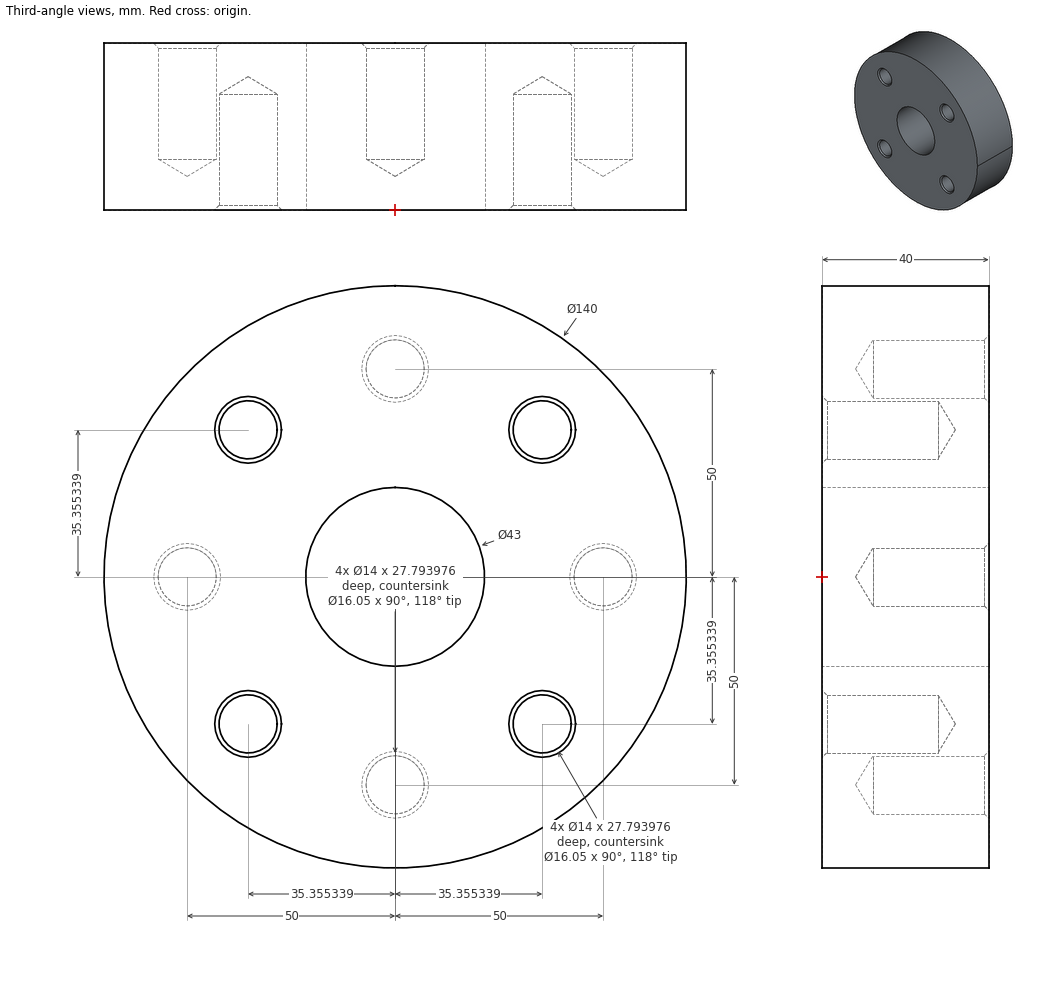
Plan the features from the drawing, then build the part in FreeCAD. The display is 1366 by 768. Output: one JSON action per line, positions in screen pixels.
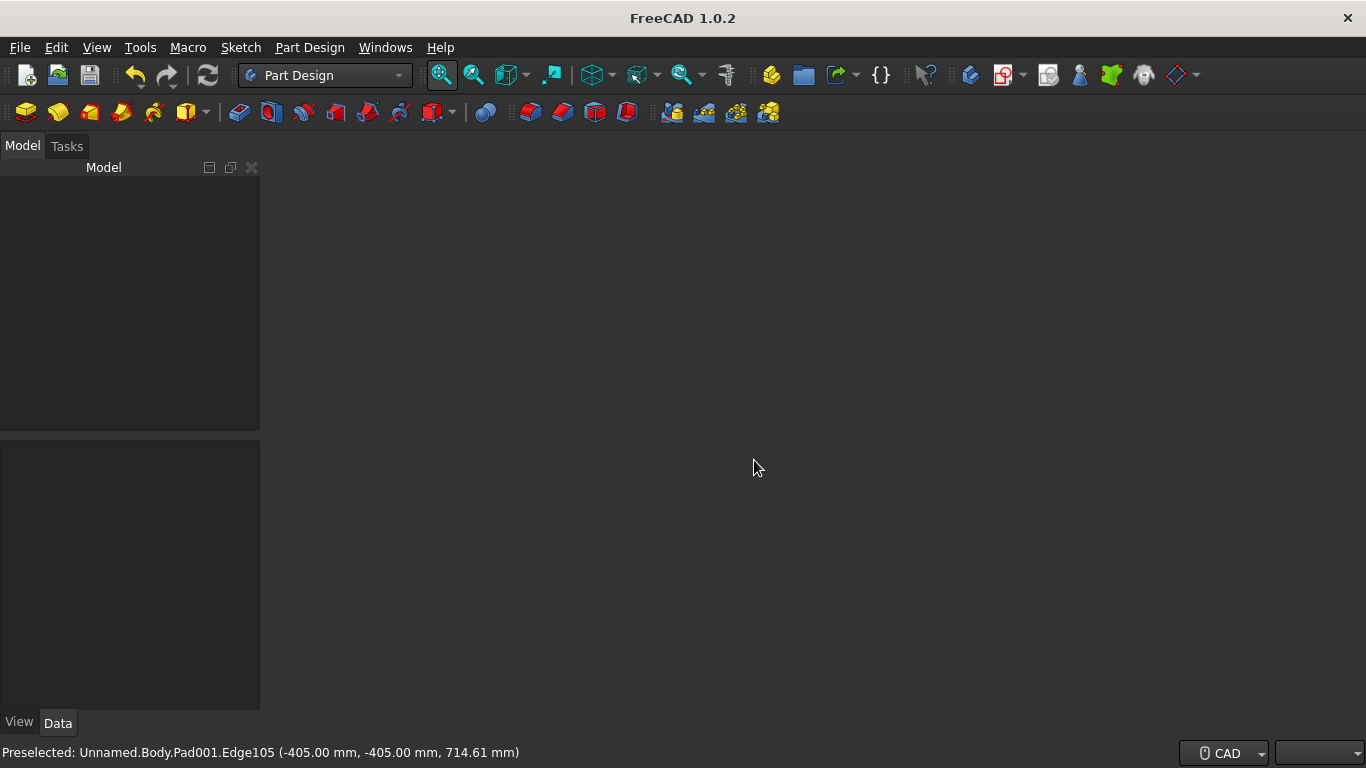
{"action": "left_click", "coordinate": [26, 76]}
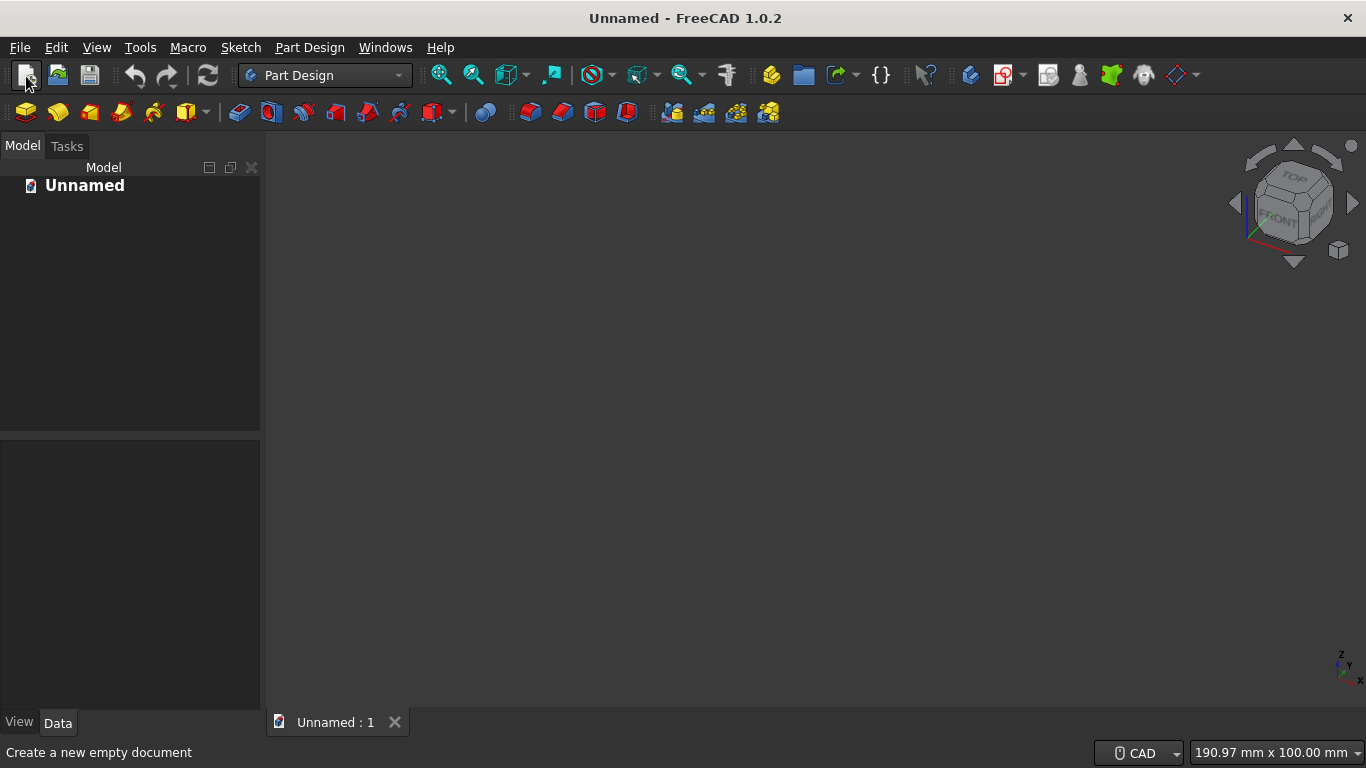
{"action": "left_click", "coordinate": [1004, 76]}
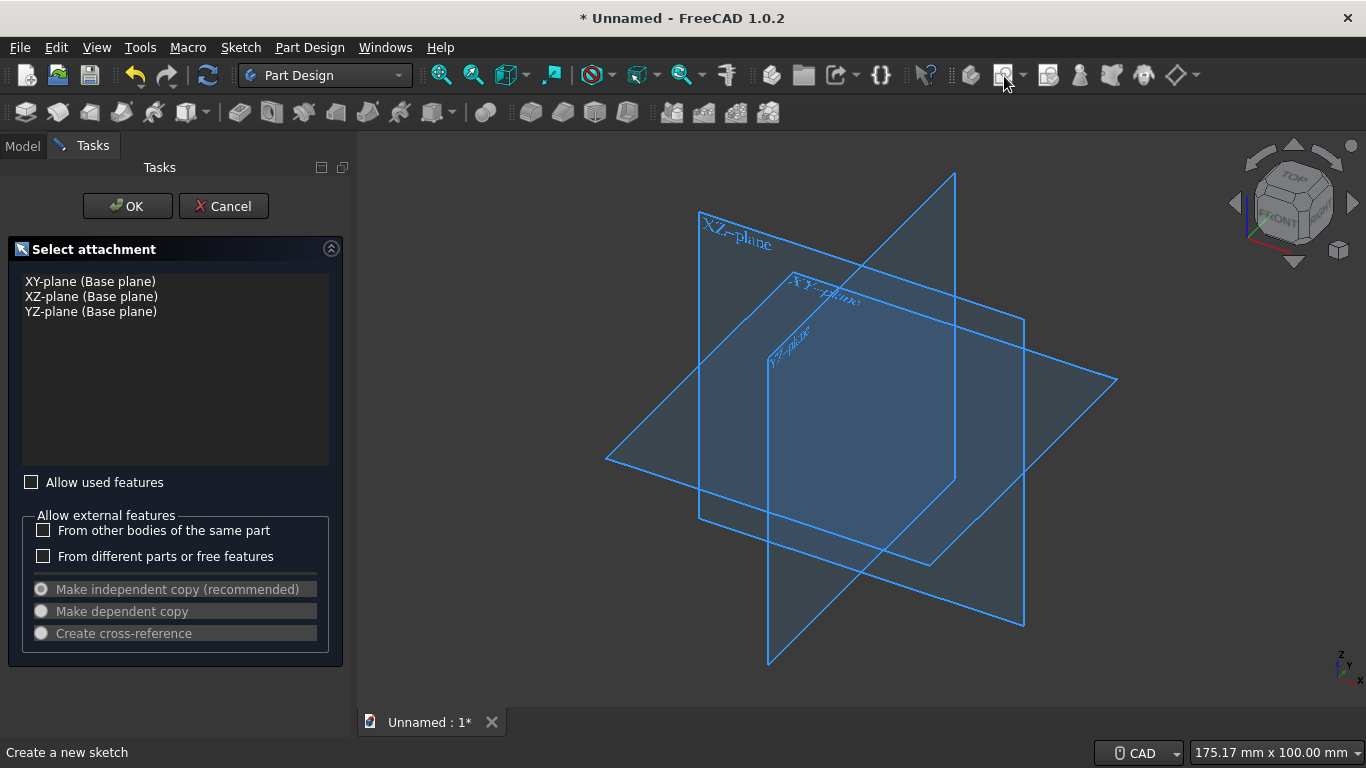
{"action": "left_click", "coordinate": [82, 296]}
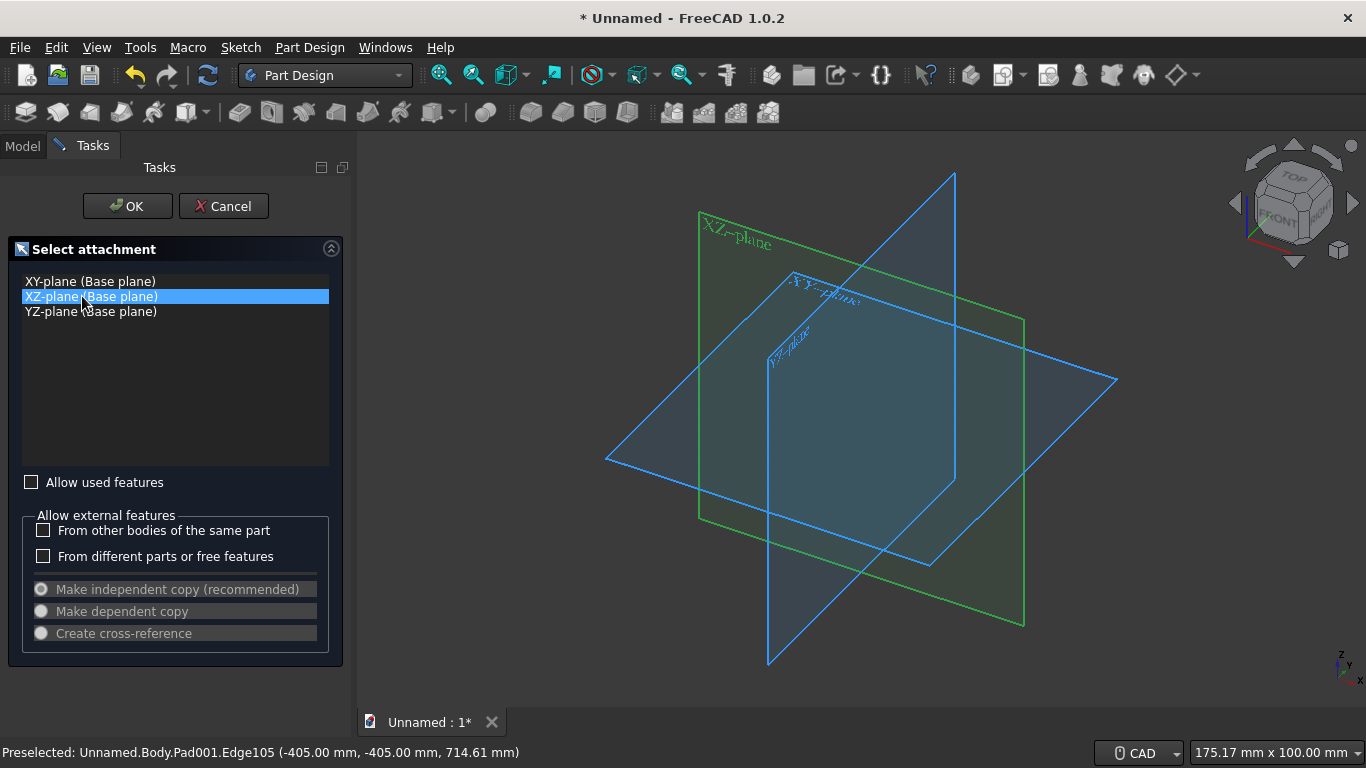
{"action": "left_click", "coordinate": [128, 206]}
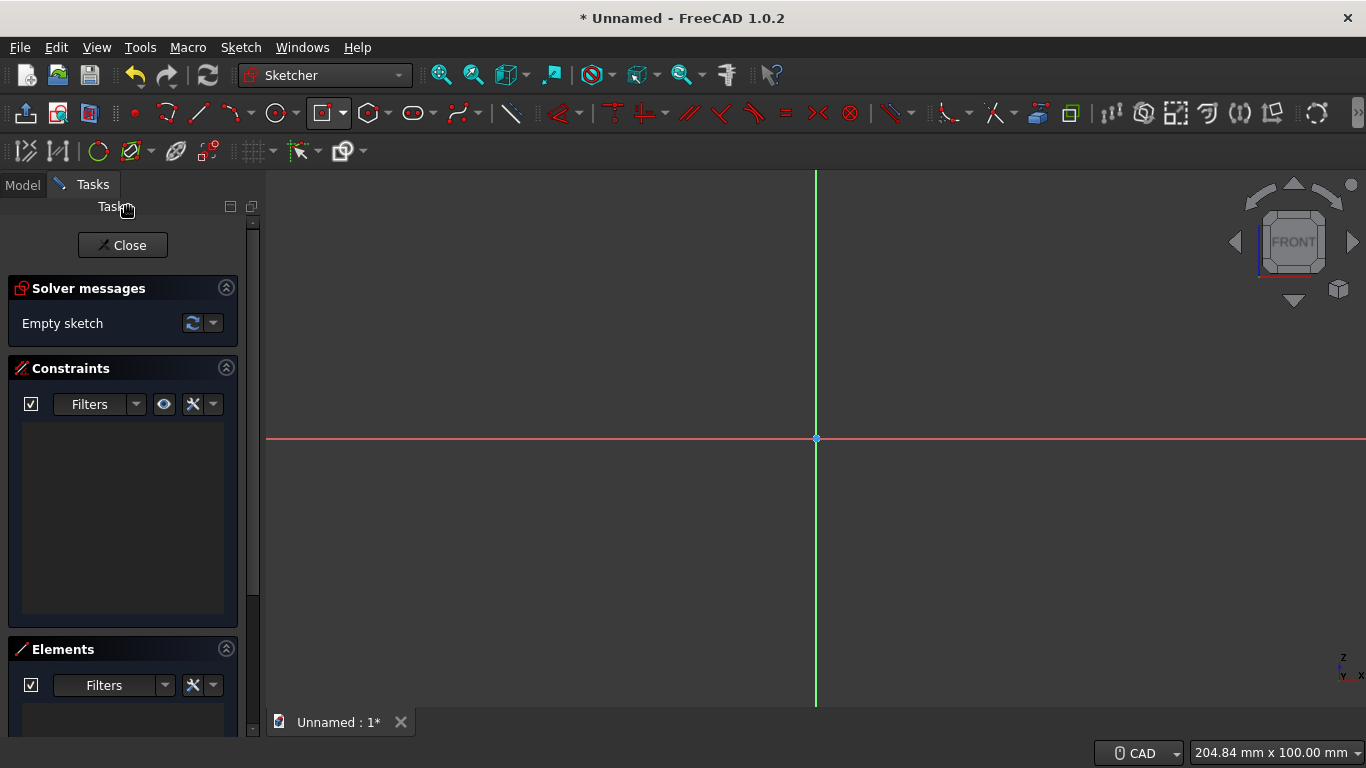
{"action": "scroll", "coordinate": [692, 438], "scroll_direction": "down", "scroll_amount": 4}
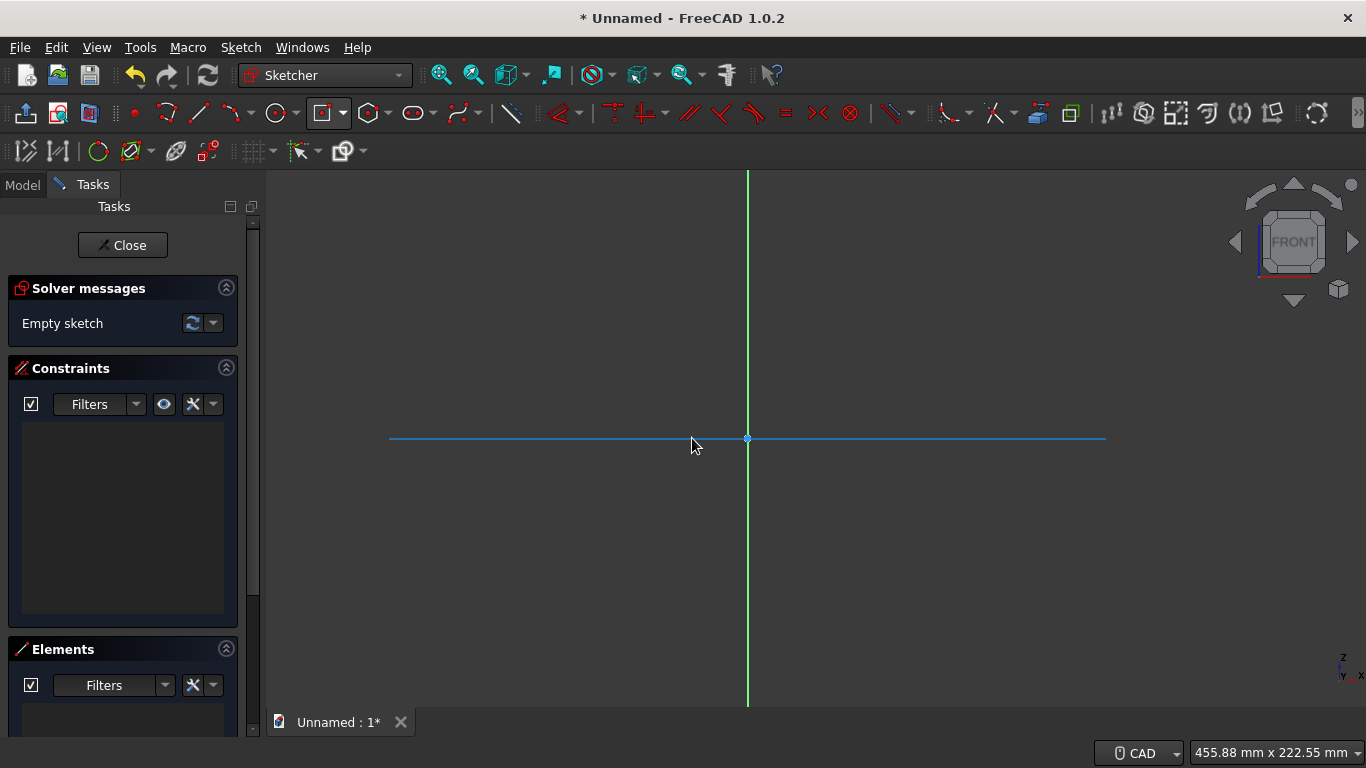
{"action": "left_click", "coordinate": [276, 114]}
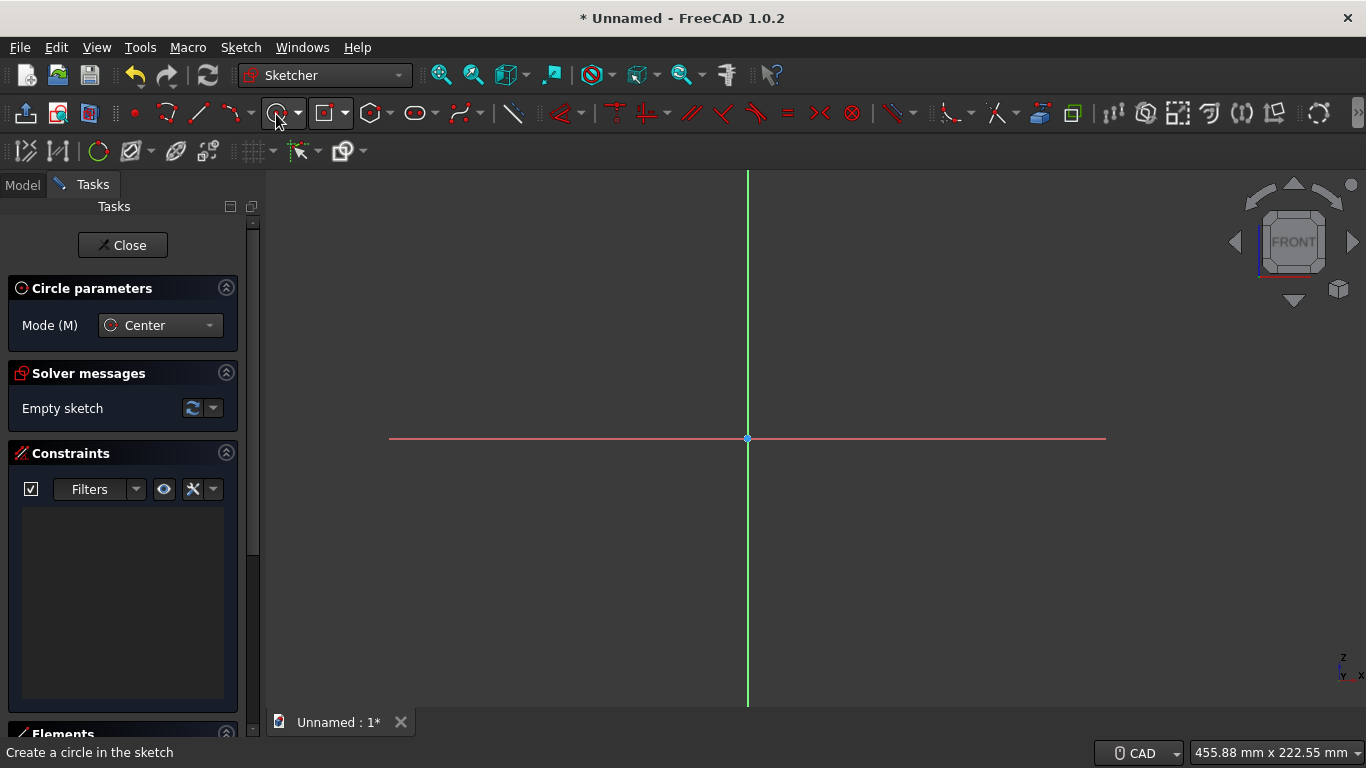
{"action": "left_click", "coordinate": [748, 438]}
{"action": "mouse_move", "coordinate": [867, 319]}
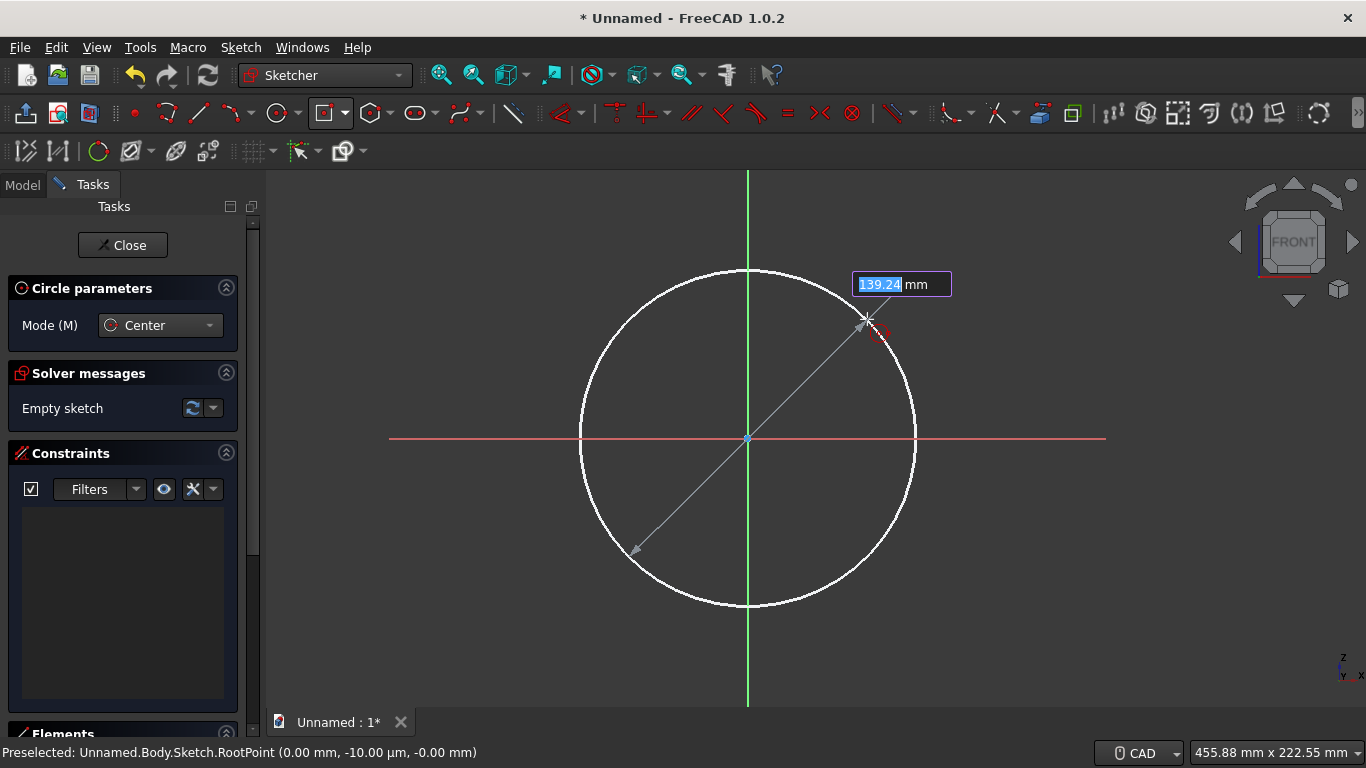
{"action": "type", "text": "140"}
{"action": "key", "text": "Return"}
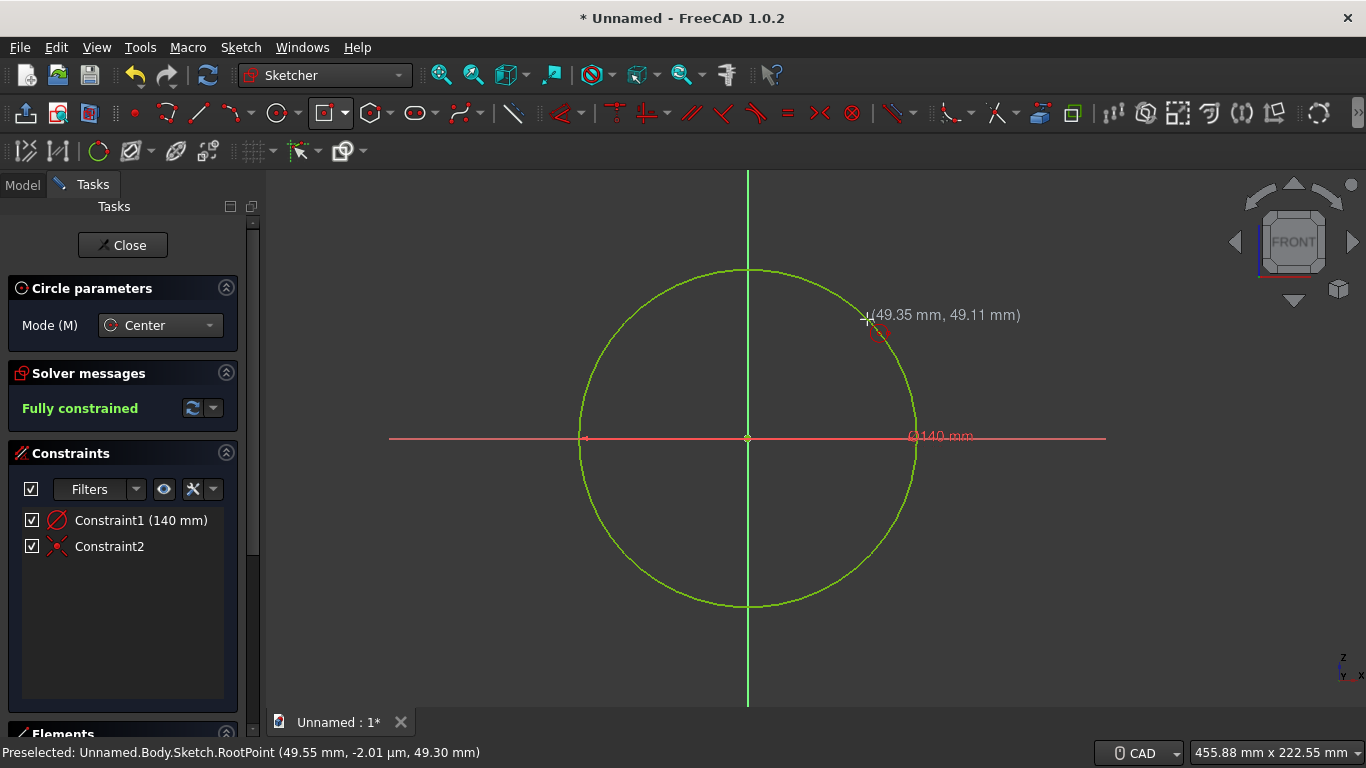
{"action": "left_click", "coordinate": [748, 438]}
{"action": "mouse_move", "coordinate": [785, 402]}